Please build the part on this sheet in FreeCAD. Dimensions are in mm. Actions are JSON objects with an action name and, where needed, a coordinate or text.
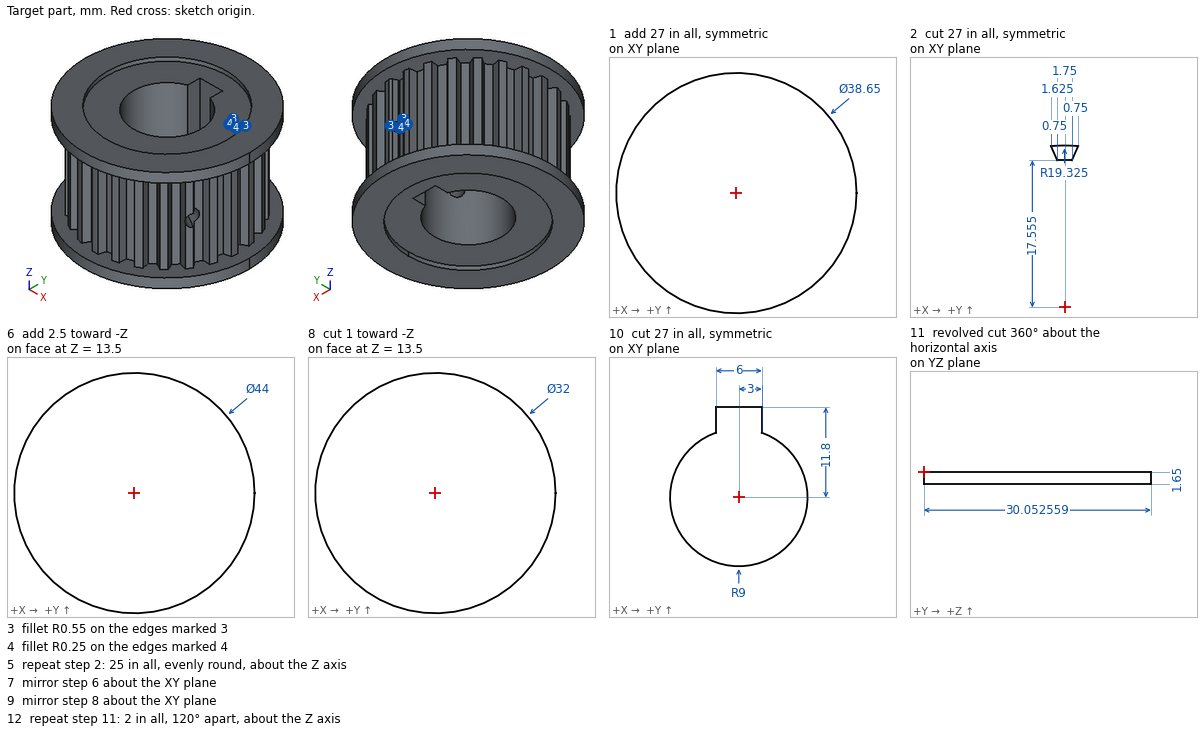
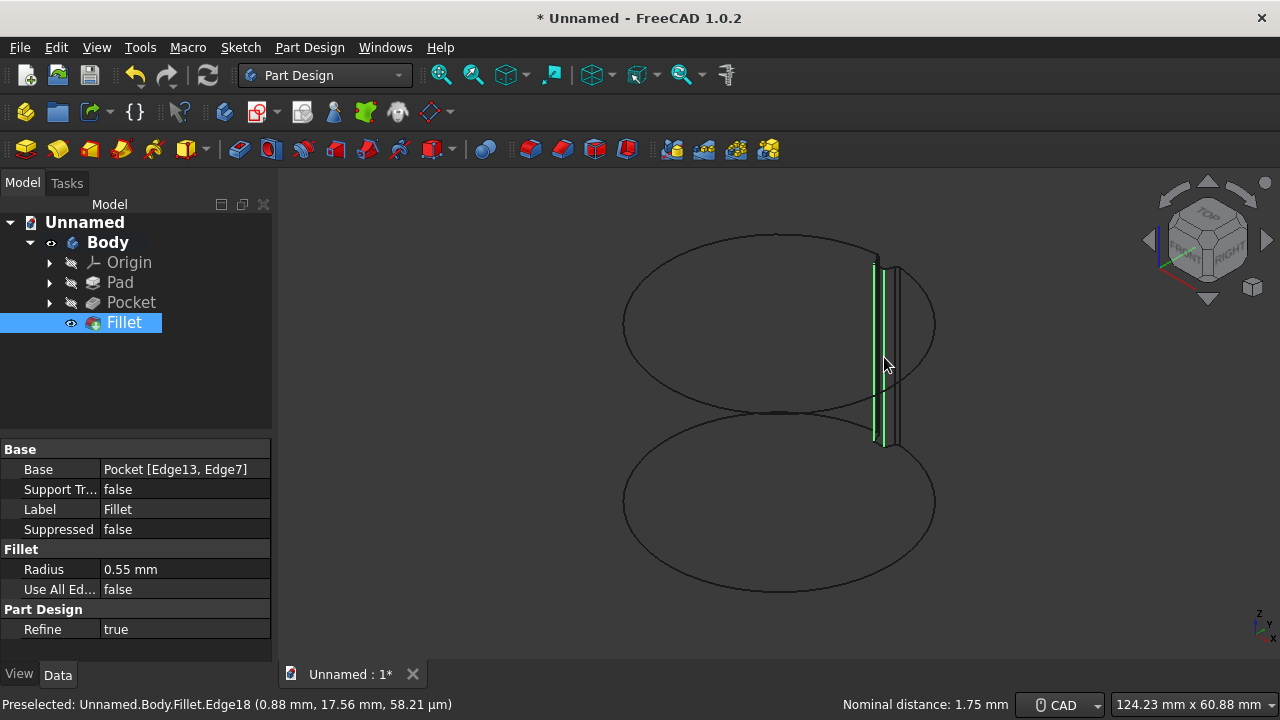
{"action": "key", "text": "v 1"}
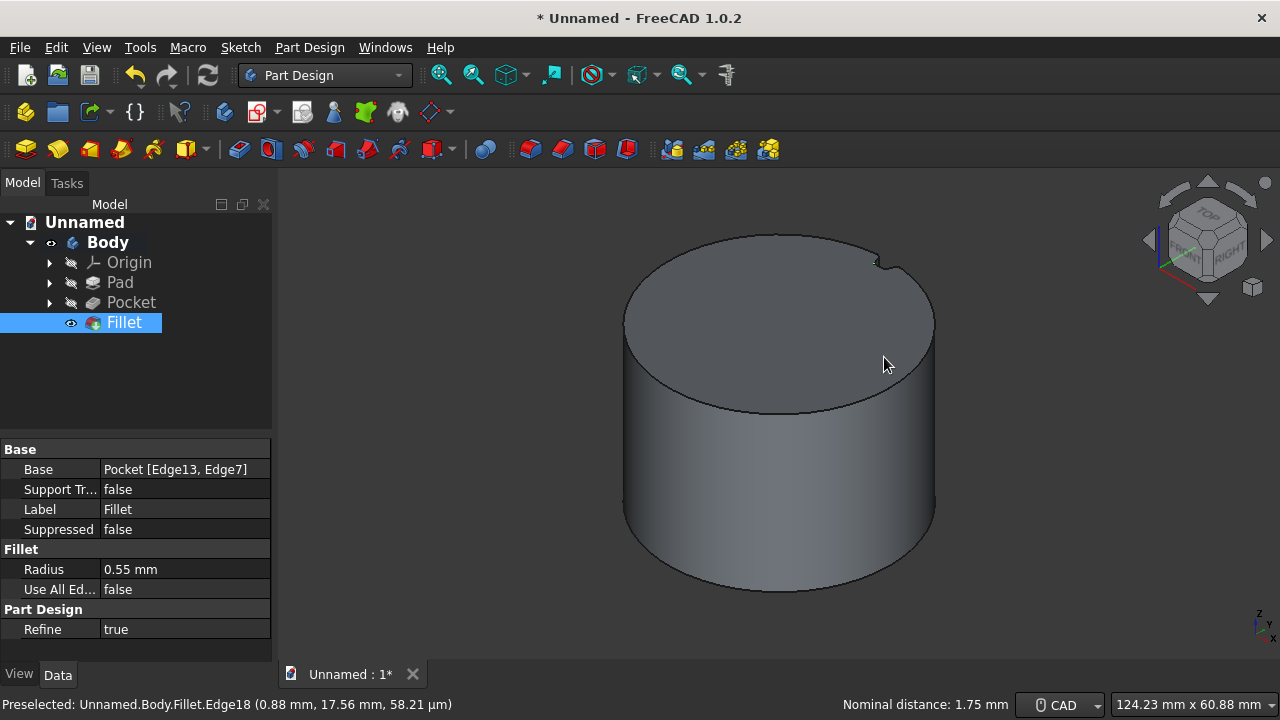
{"action": "left_click", "coordinate": [532, 150]}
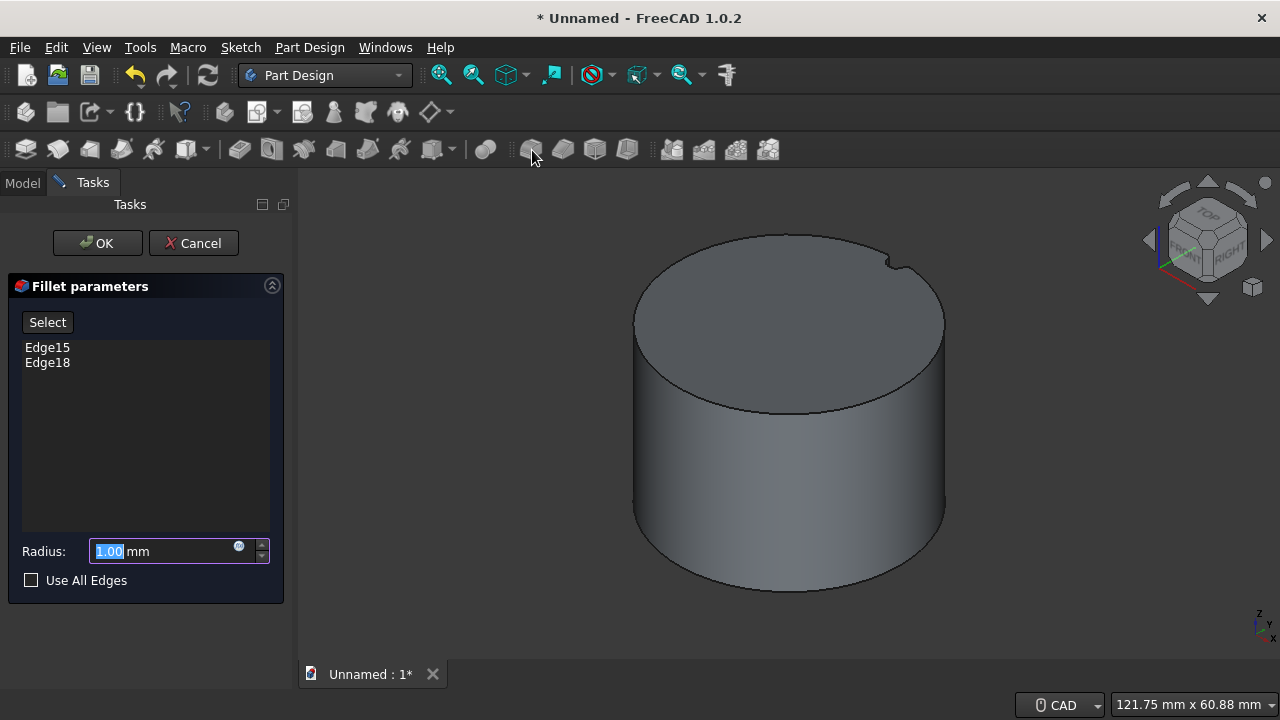
{"action": "type", "text": "0.25"}
{"action": "key", "text": "Tab"}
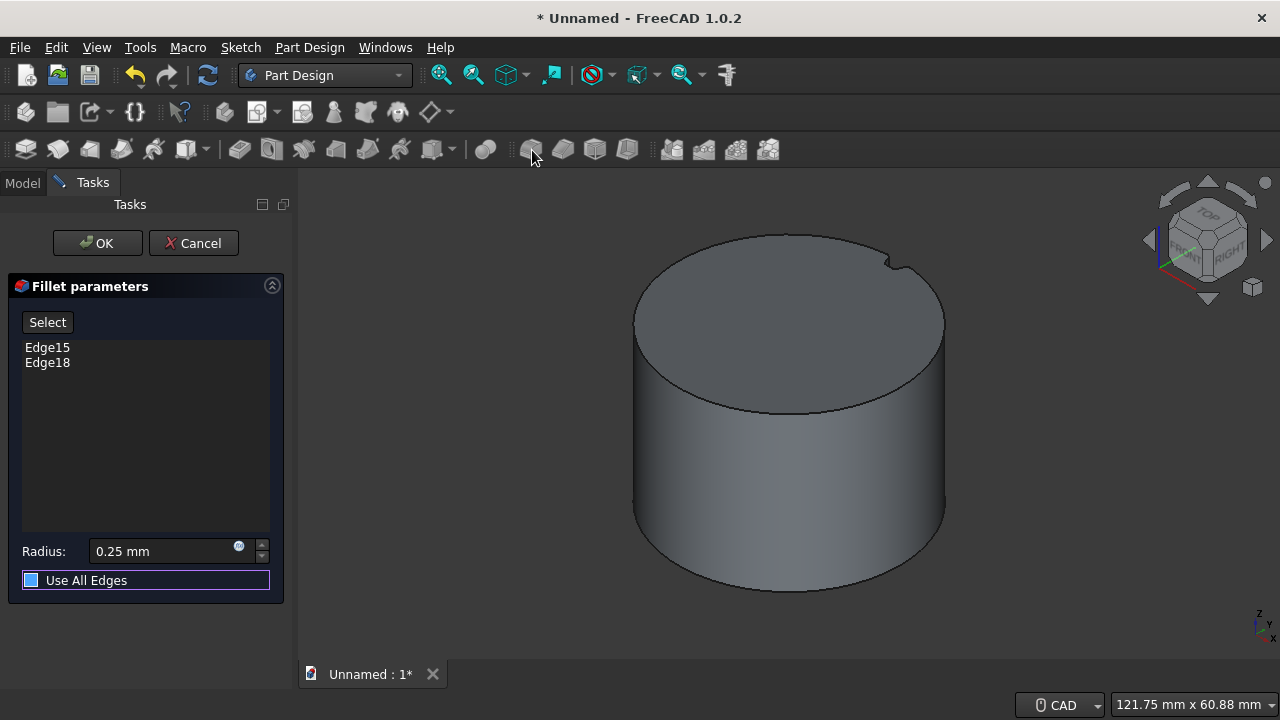
{"action": "left_click", "coordinate": [98, 243]}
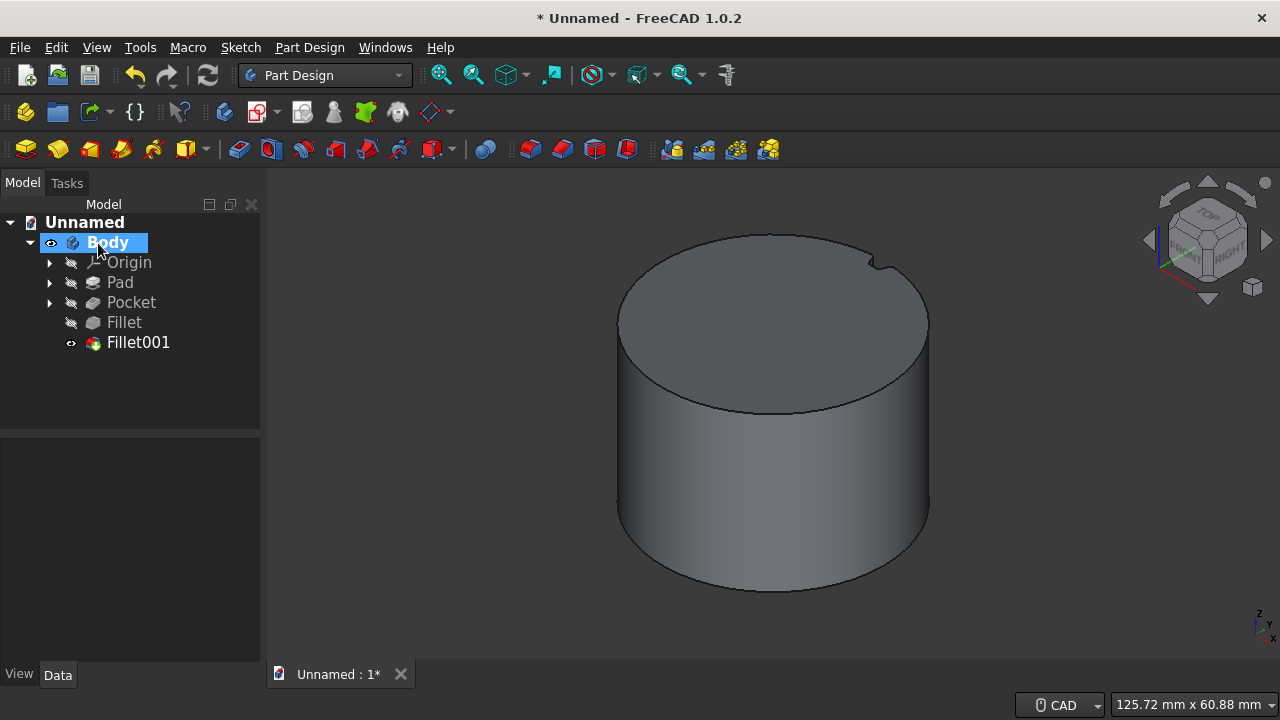
{"action": "left_click", "coordinate": [116, 303]}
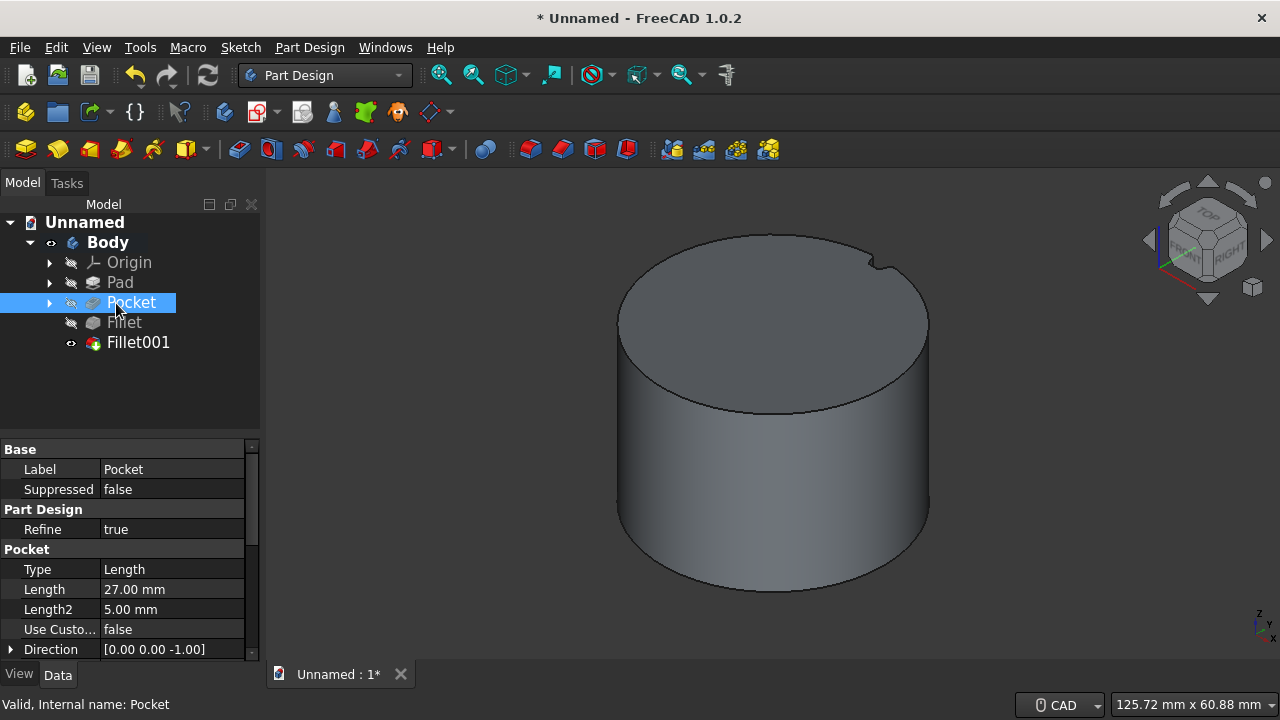
{"action": "left_click", "coordinate": [736, 150]}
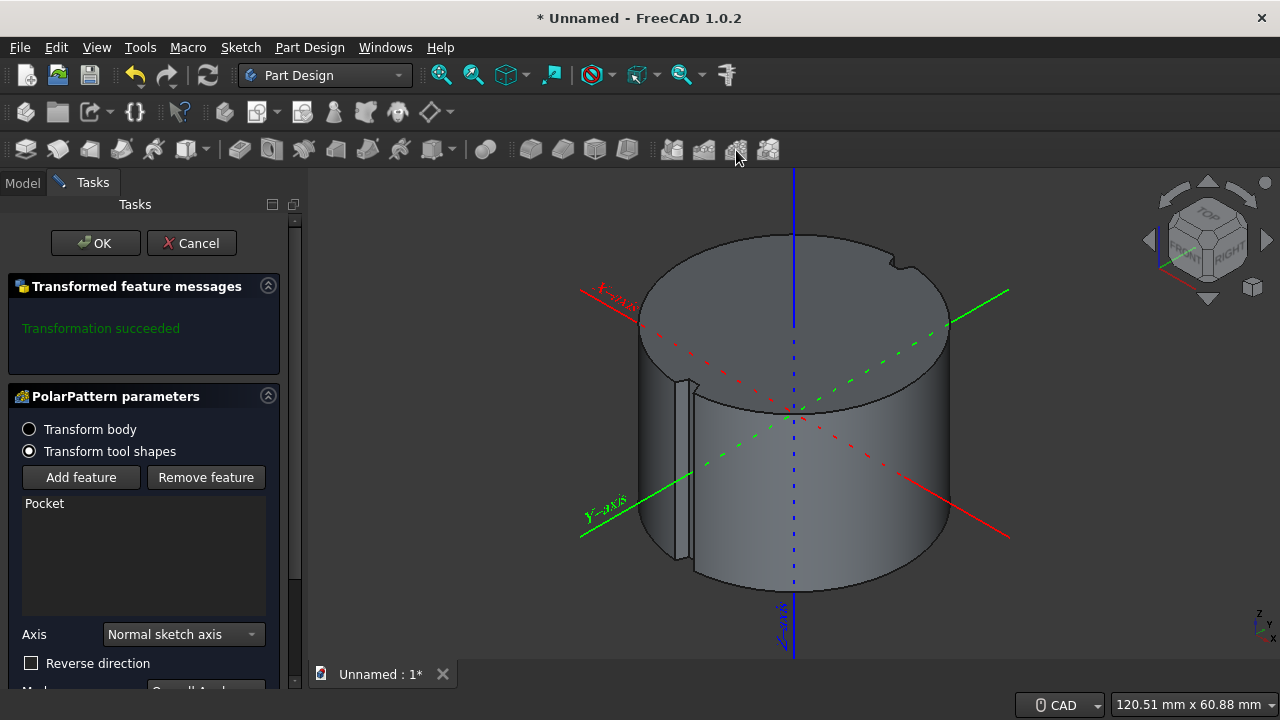
{"action": "left_click", "coordinate": [184, 634]}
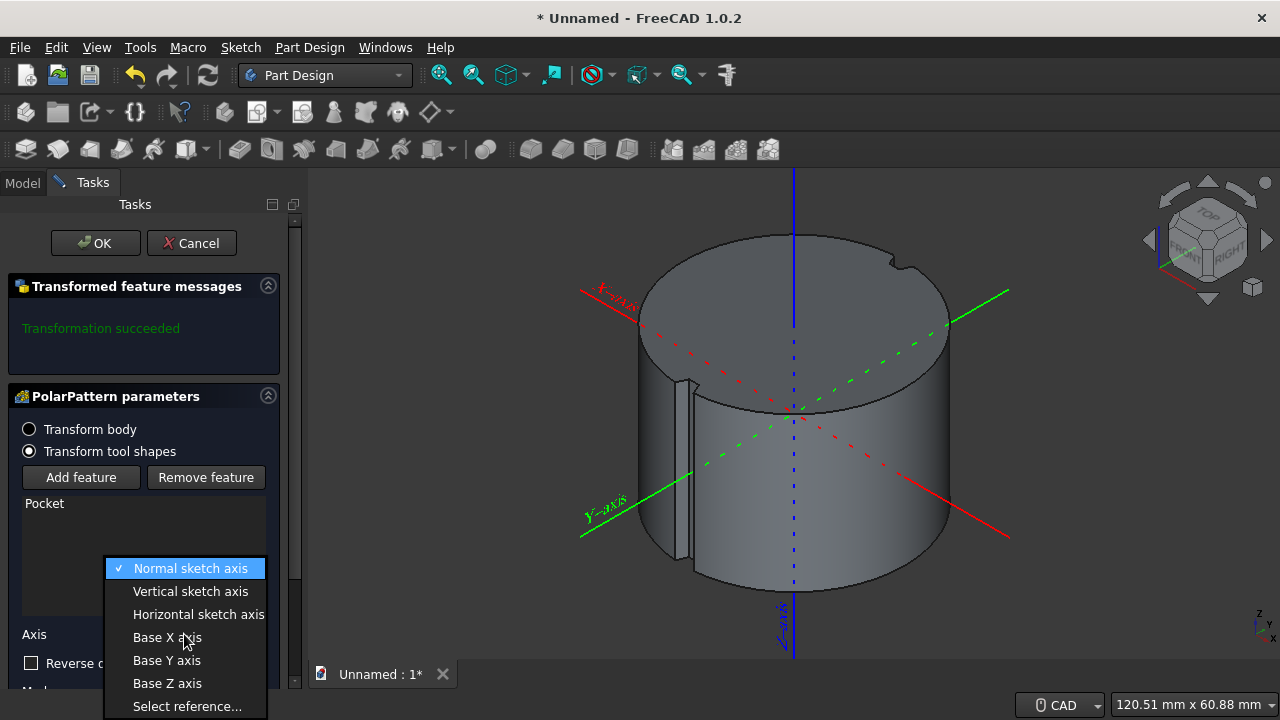
{"action": "left_click", "coordinate": [184, 684]}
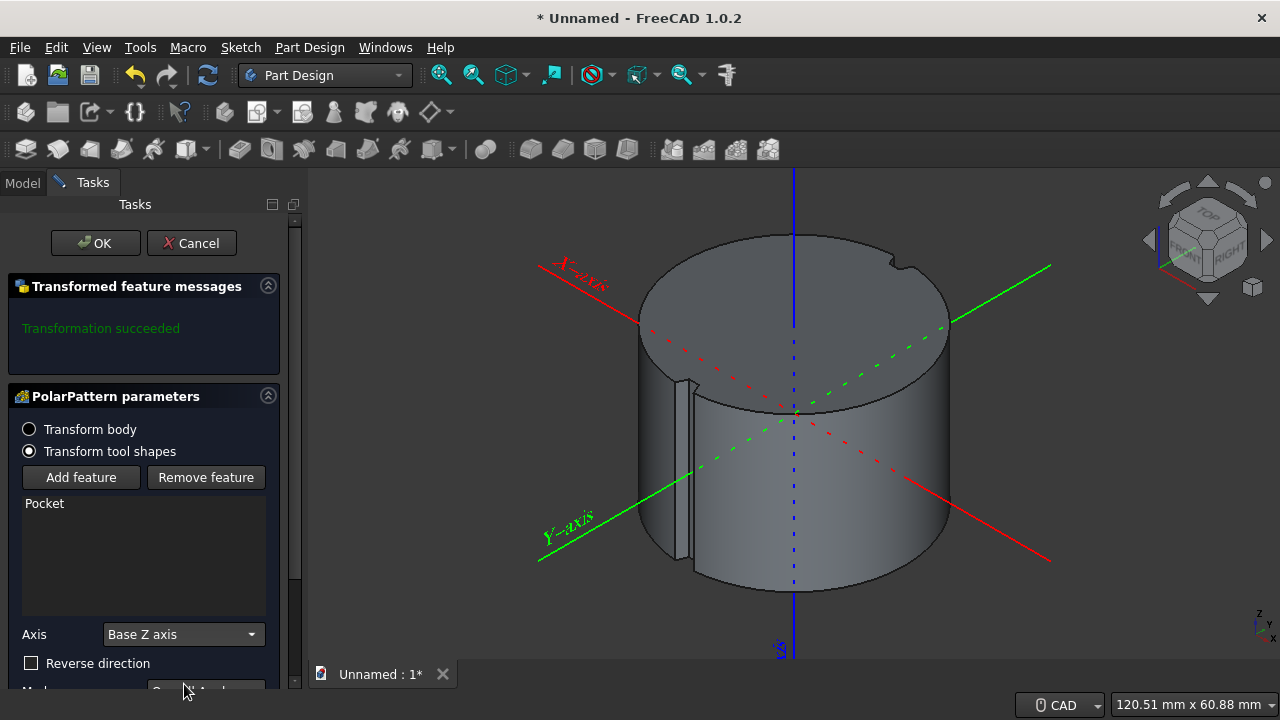
{"action": "scroll", "coordinate": [295, 451], "scroll_direction": "down", "scroll_amount": 3}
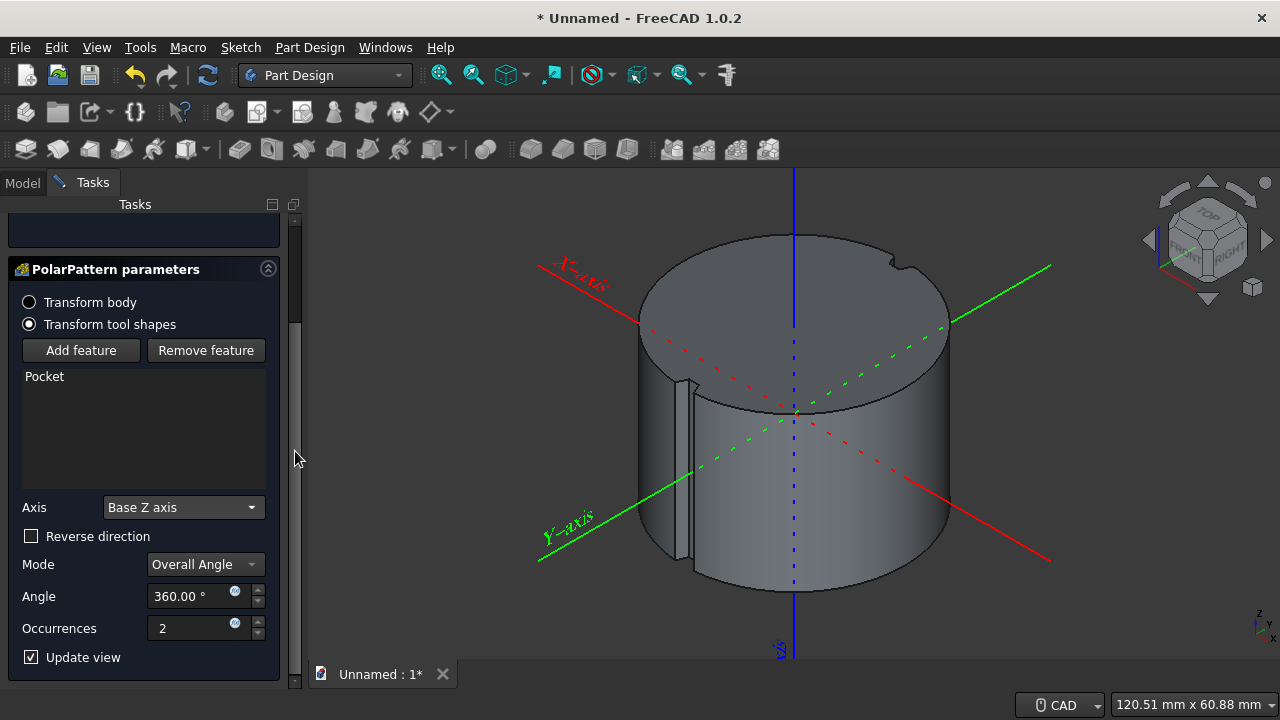
{"action": "triple_click", "coordinate": [198, 628]}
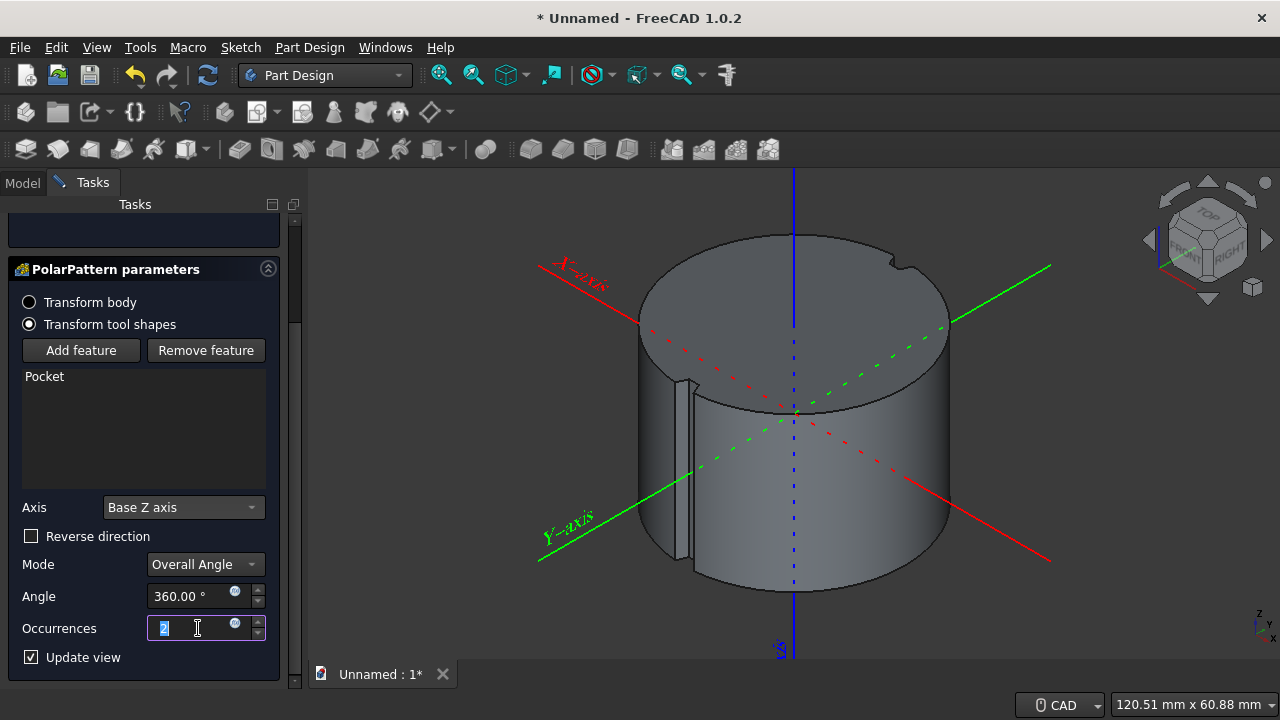
{"action": "type", "text": "25"}
{"action": "key", "text": "Tab"}